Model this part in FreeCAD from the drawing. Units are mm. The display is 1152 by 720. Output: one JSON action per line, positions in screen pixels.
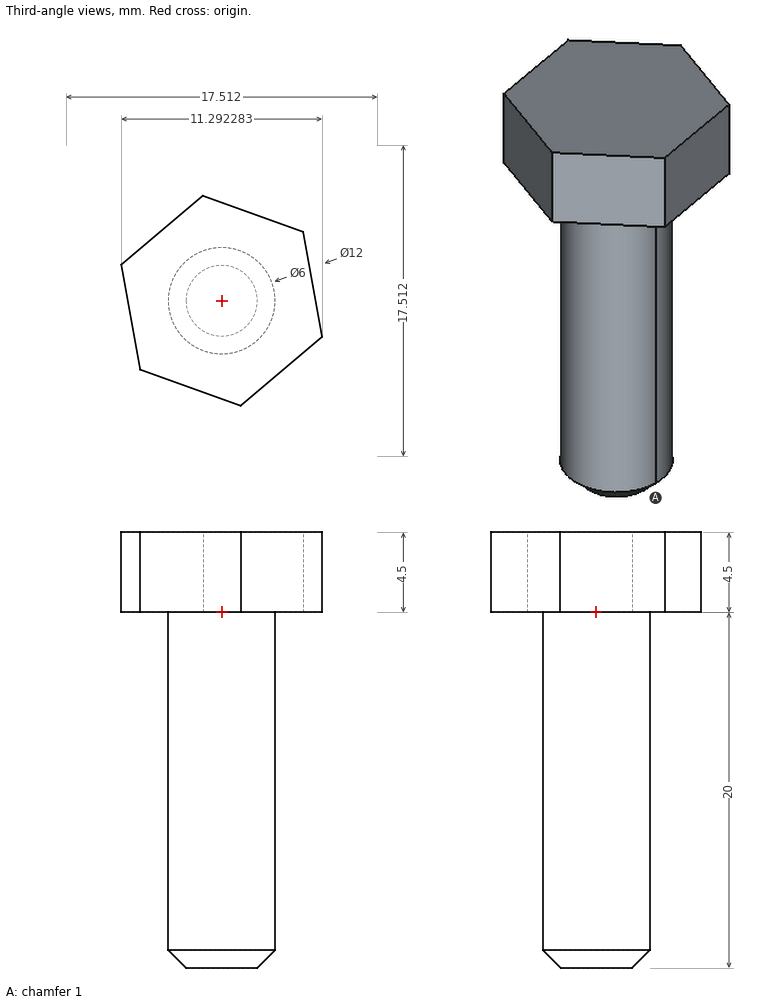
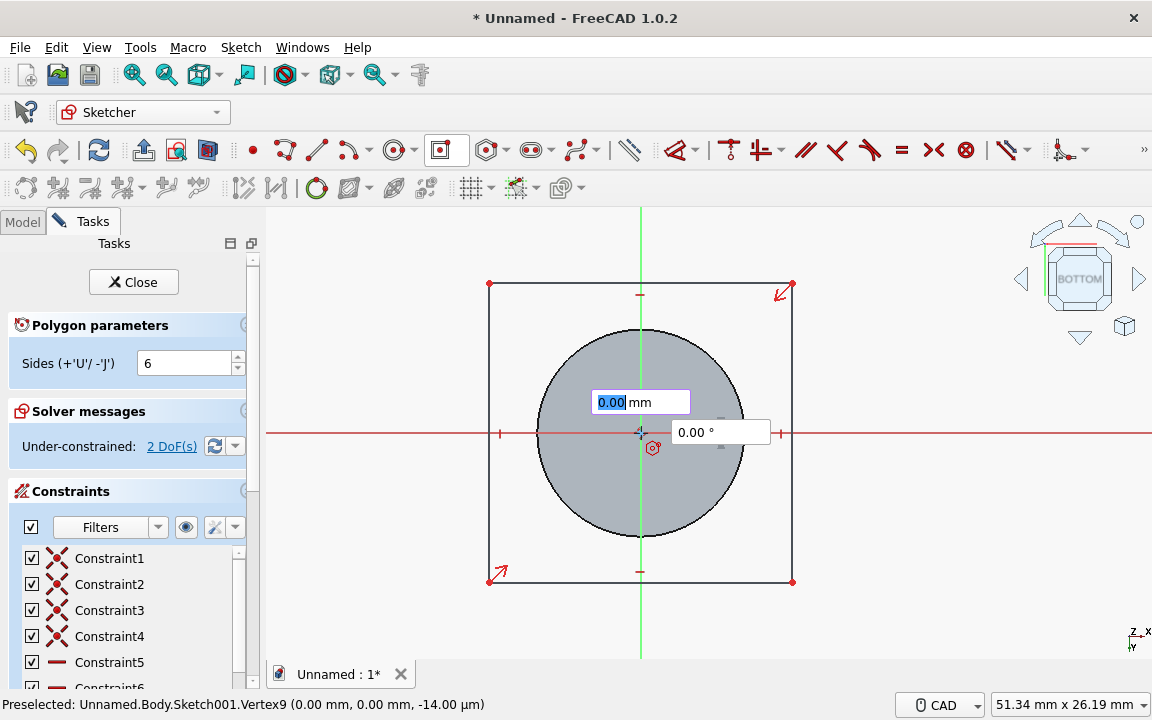
{"action": "left_click", "coordinate": [562, 366]}
{"action": "right_click", "coordinate": [562, 366]}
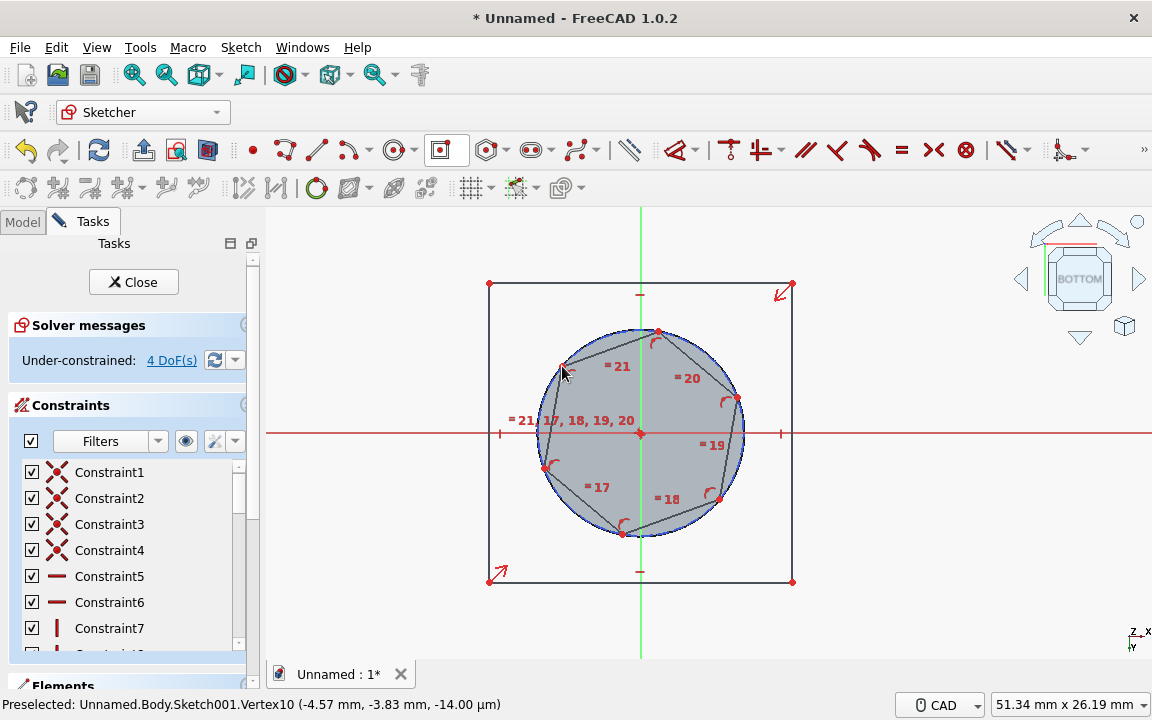
{"action": "left_click", "coordinate": [676, 150]}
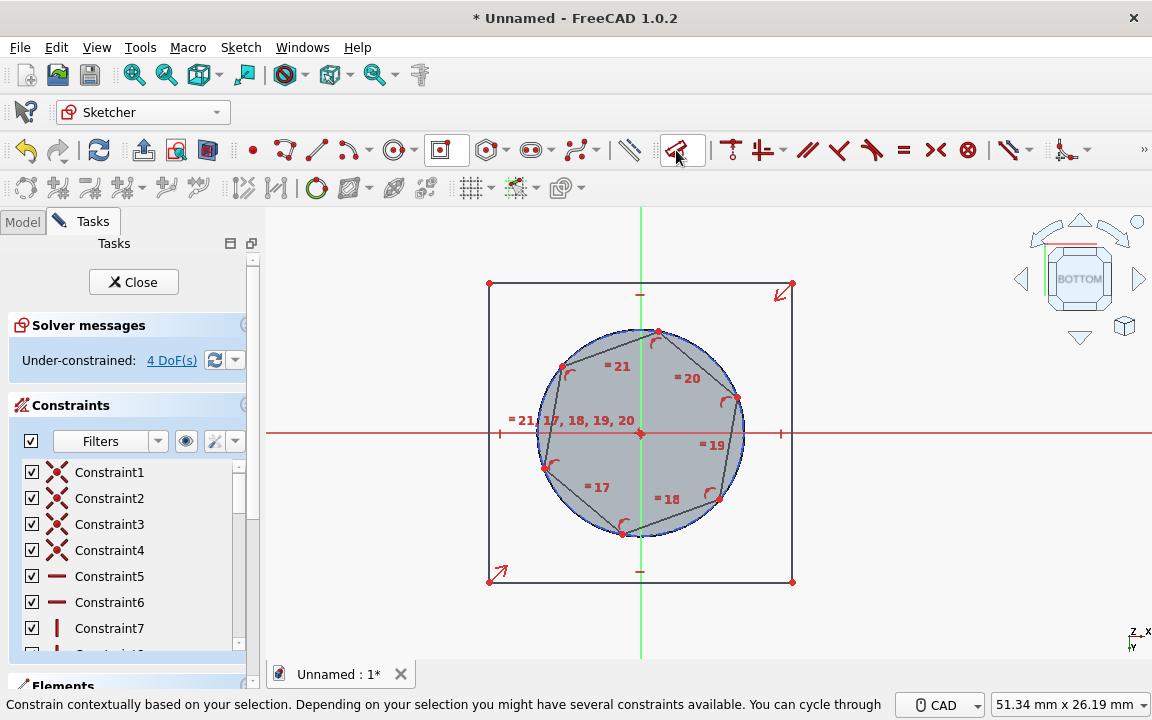
{"action": "left_click", "coordinate": [713, 360]}
{"action": "left_click", "coordinate": [735, 337]}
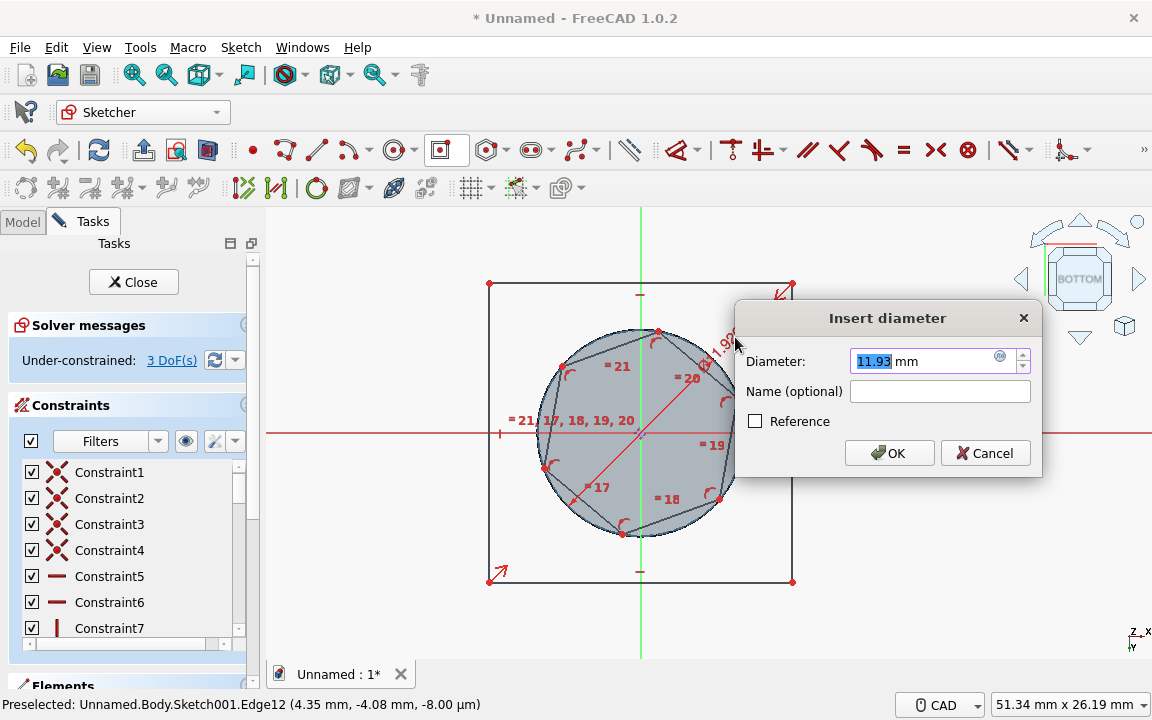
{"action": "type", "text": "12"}
{"action": "key", "text": "Return"}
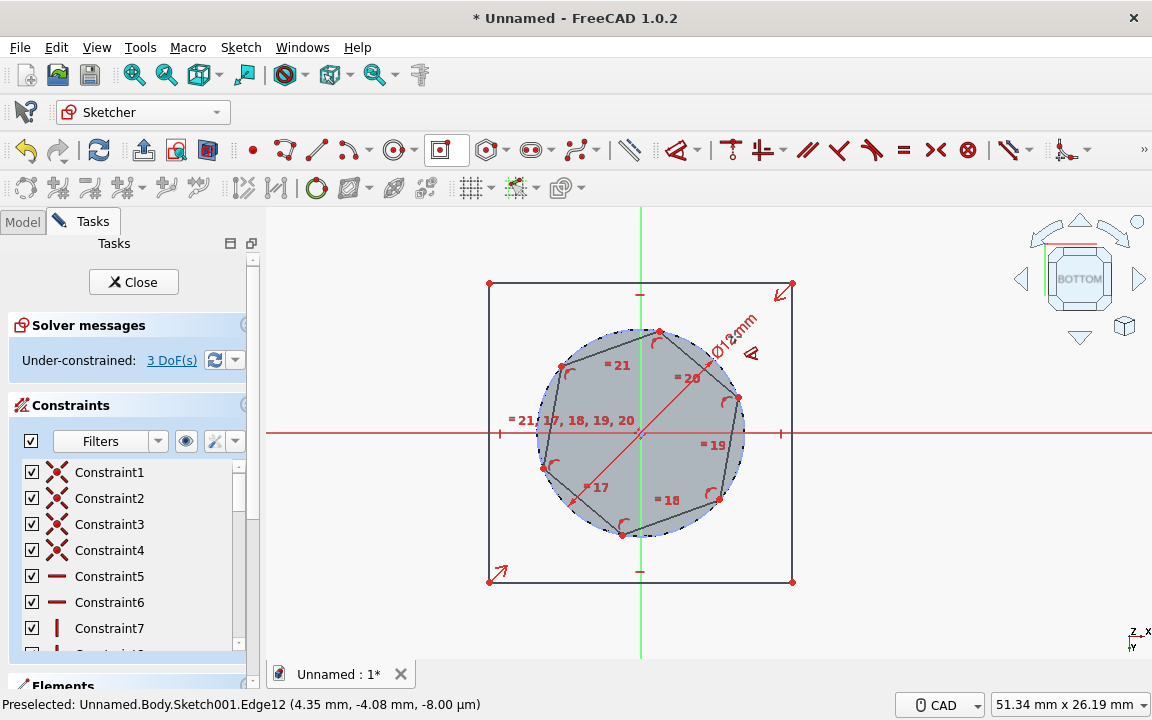
{"action": "left_click", "coordinate": [580, 583]}
{"action": "left_click", "coordinate": [571, 617]}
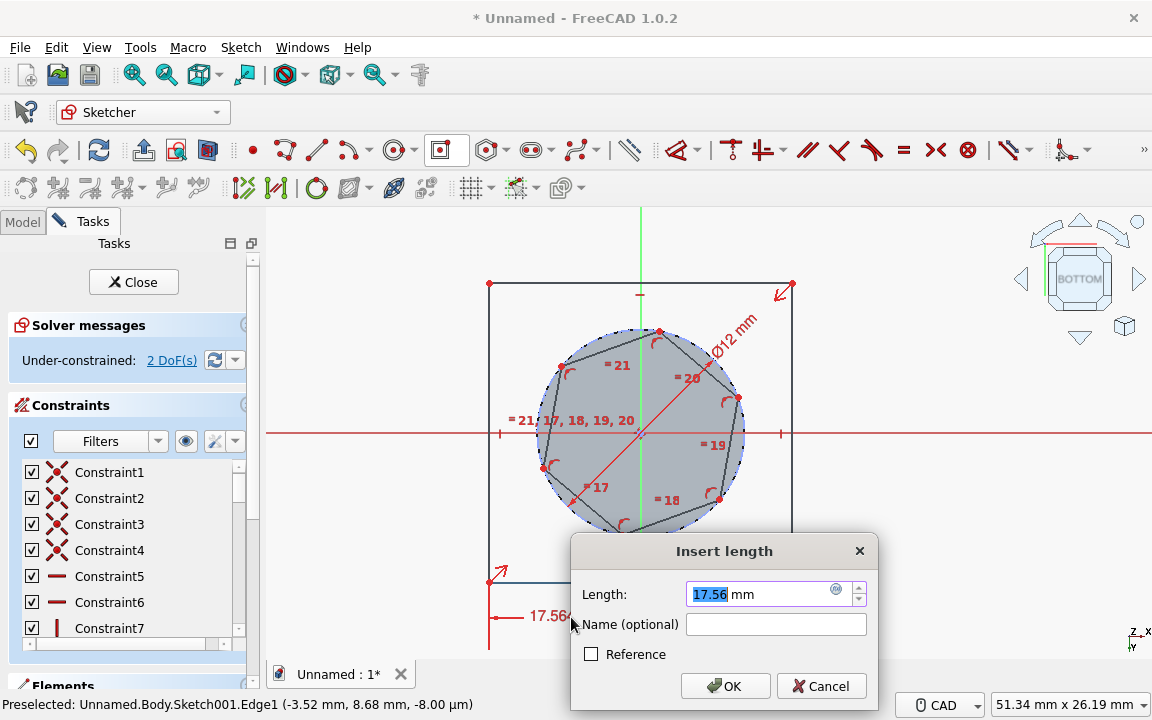
{"action": "type", "text": "17.512"}
{"action": "key", "text": "Return"}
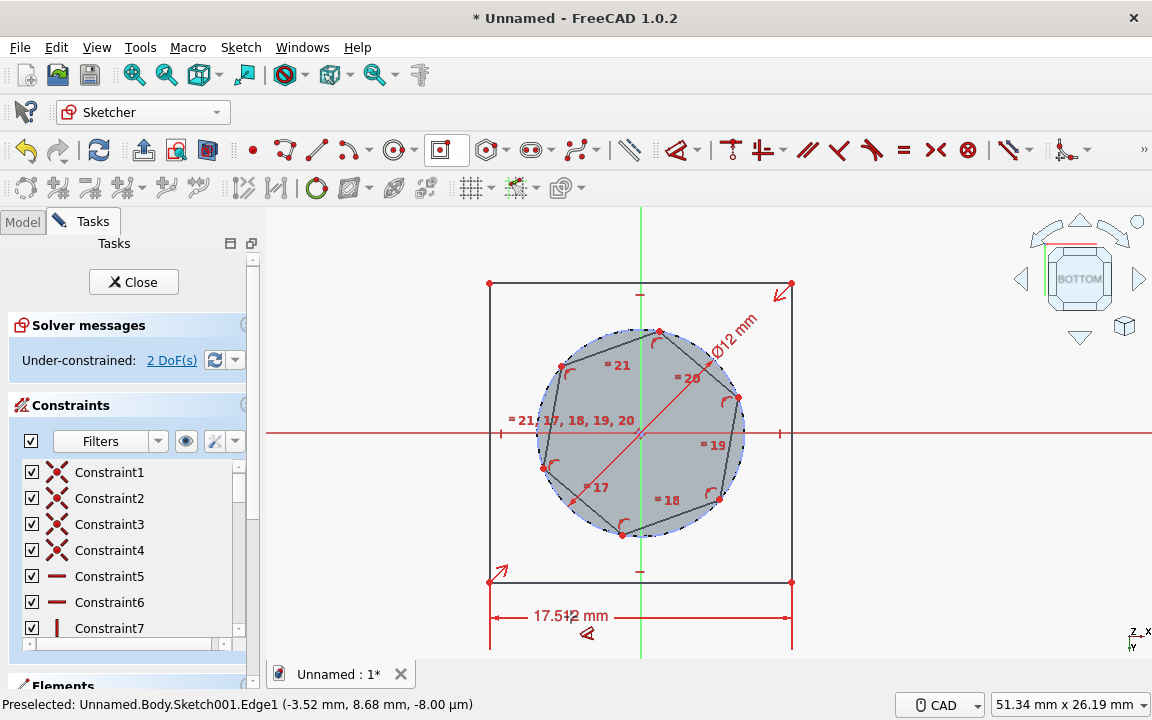
{"action": "left_click", "coordinate": [792, 493]}
{"action": "left_click", "coordinate": [826, 364]}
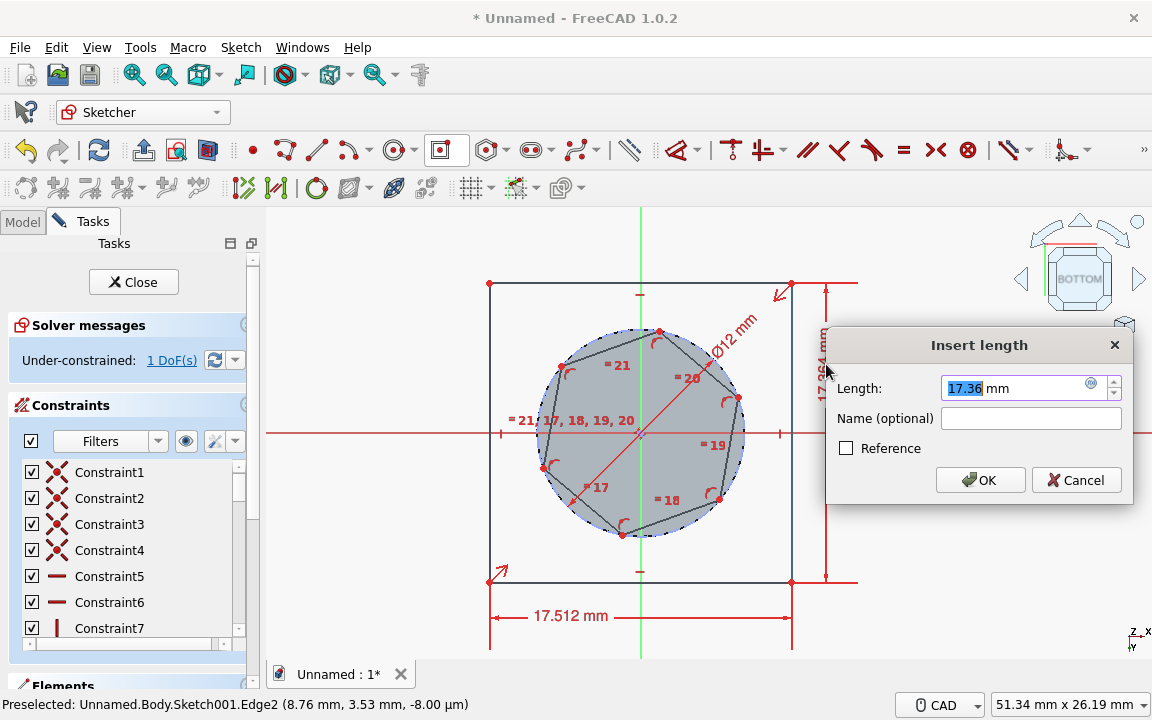
{"action": "type", "text": "17.512"}
{"action": "key", "text": "Return"}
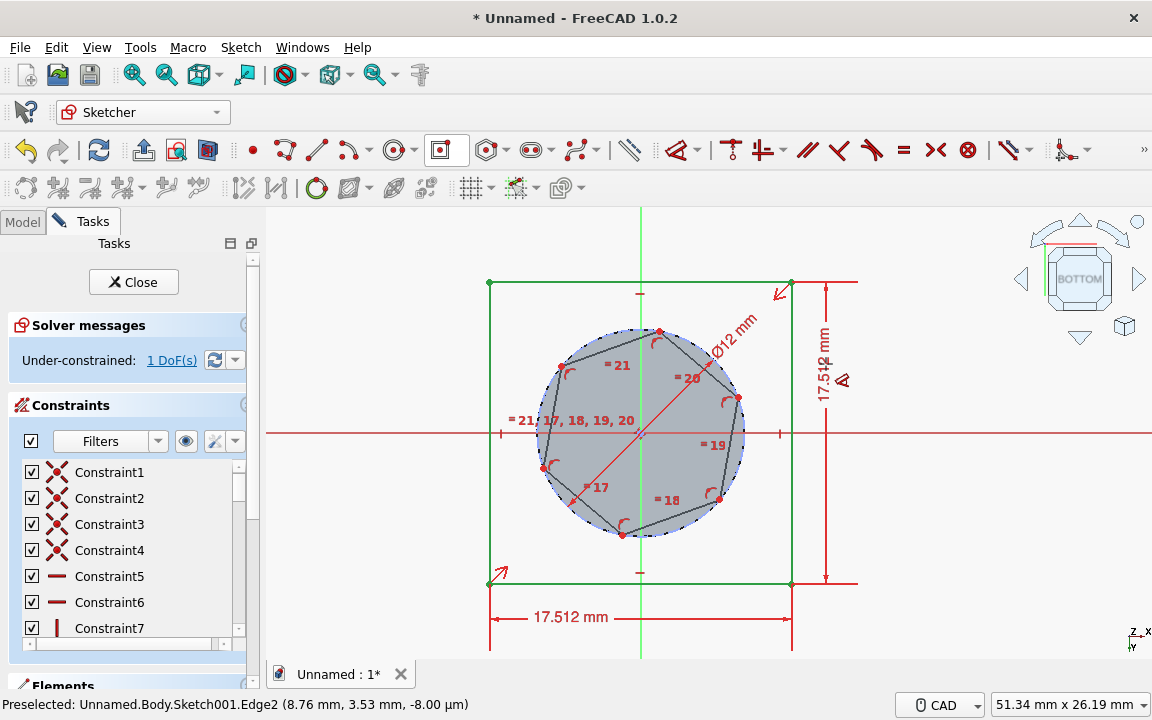
{"action": "left_click", "coordinate": [543, 468]}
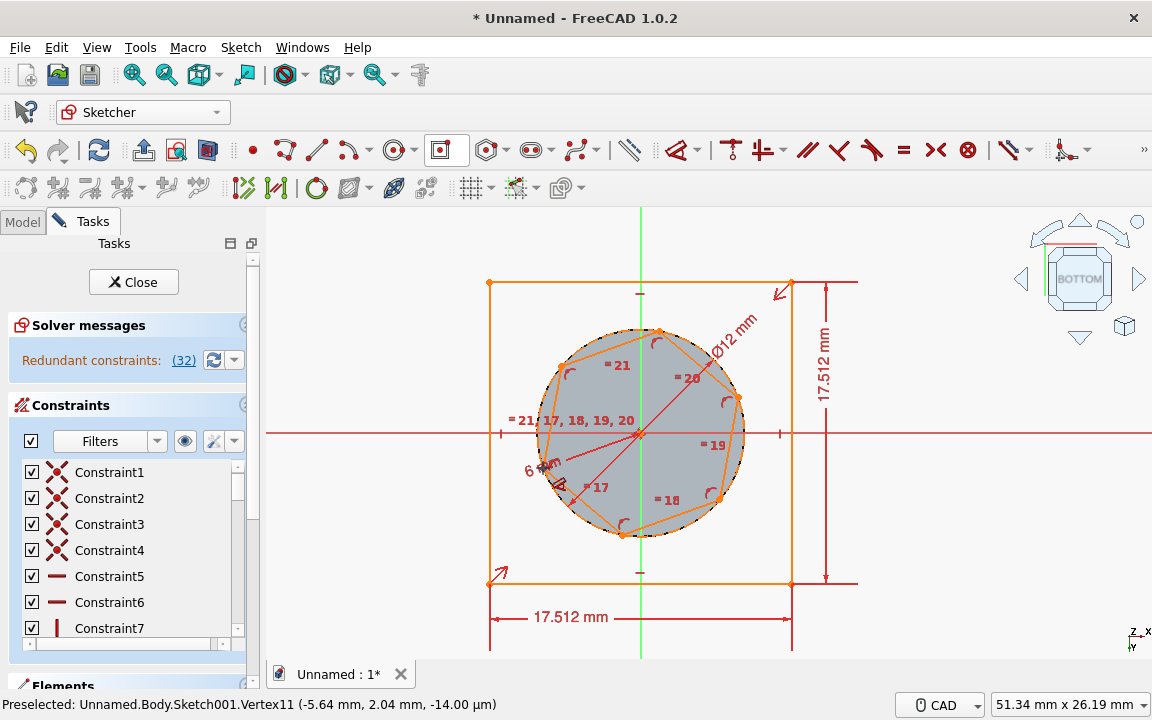
{"action": "left_click", "coordinate": [738, 398]}
{"action": "left_click", "coordinate": [596, 550]}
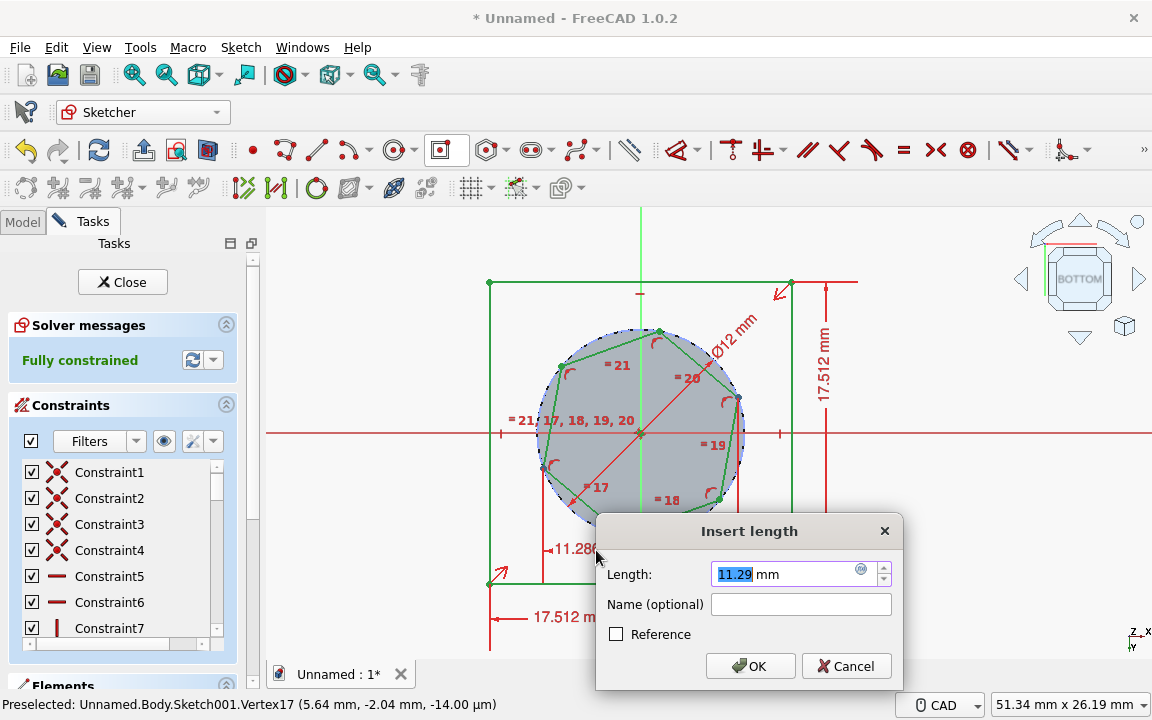
{"action": "type", "text": "11.292283"}
{"action": "key", "text": "Return"}
{"action": "key", "text": "Escape"}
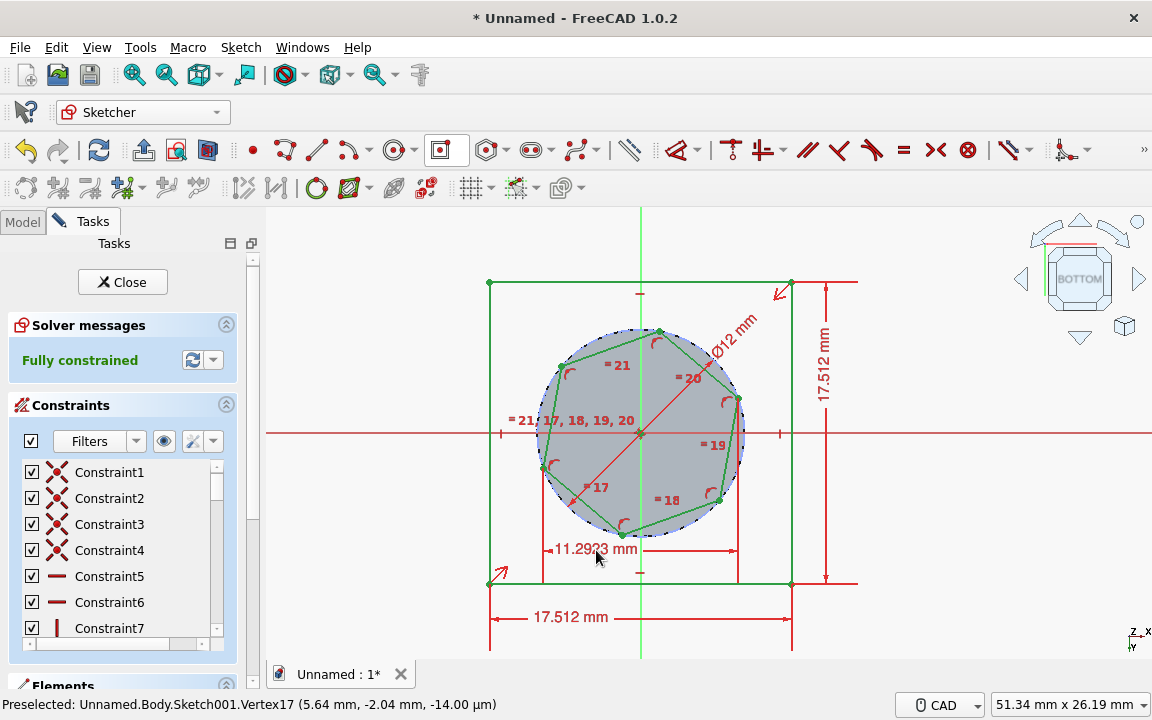
{"action": "left_click", "coordinate": [123, 282]}